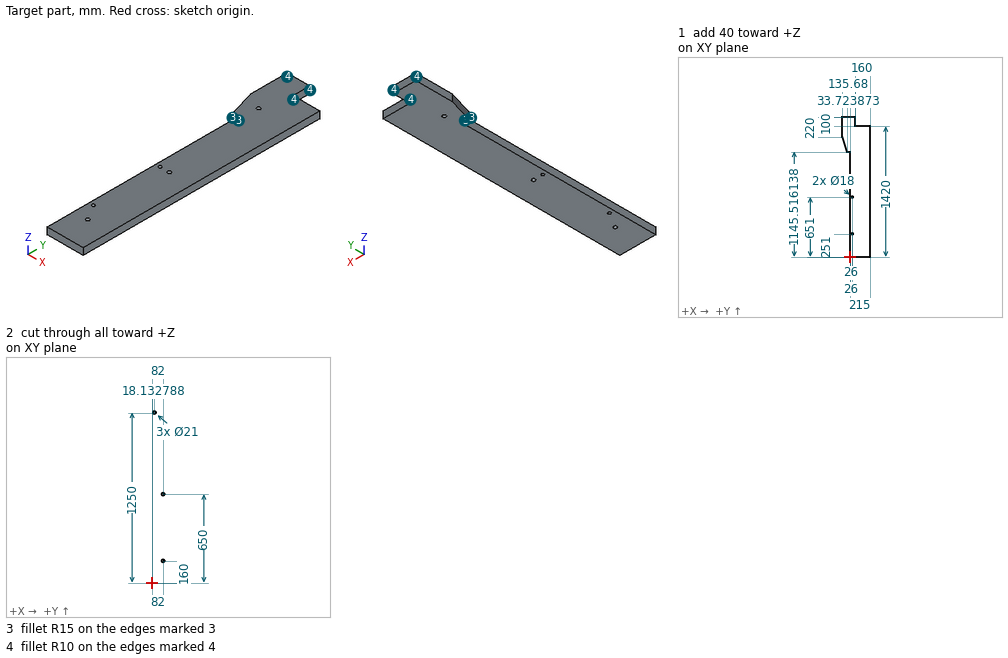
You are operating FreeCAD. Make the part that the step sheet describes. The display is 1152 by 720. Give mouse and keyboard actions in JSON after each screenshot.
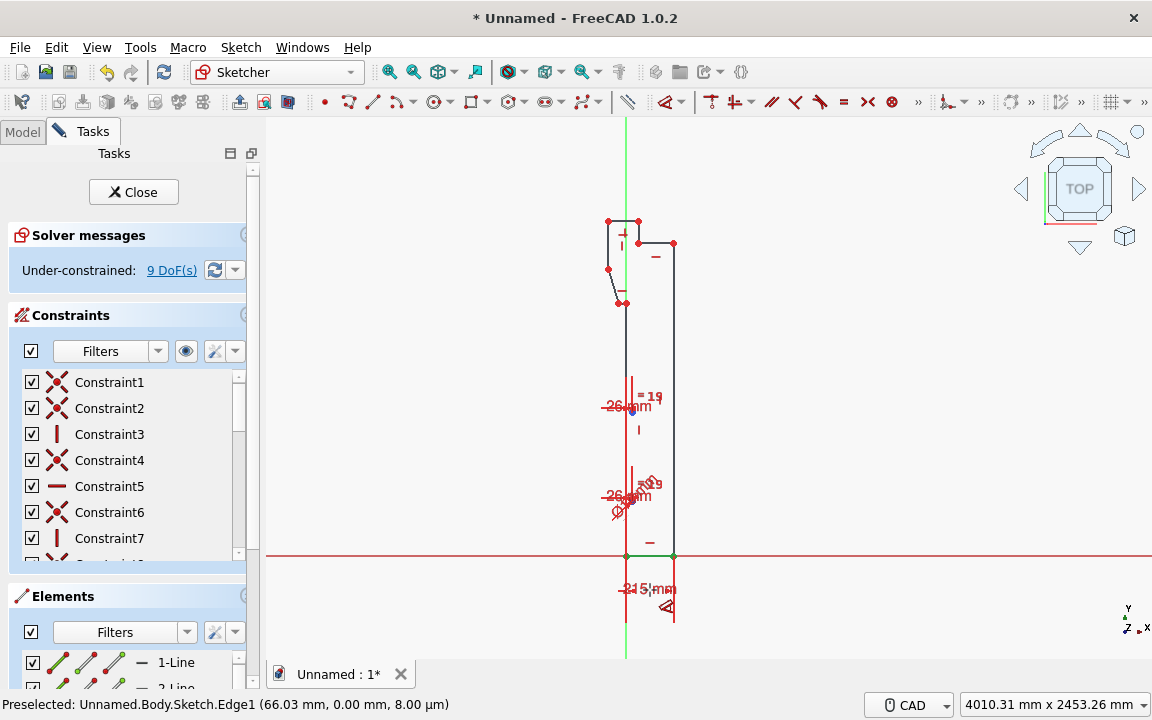
{"action": "scroll", "coordinate": [663, 243], "scroll_direction": "up", "scroll_amount": 2}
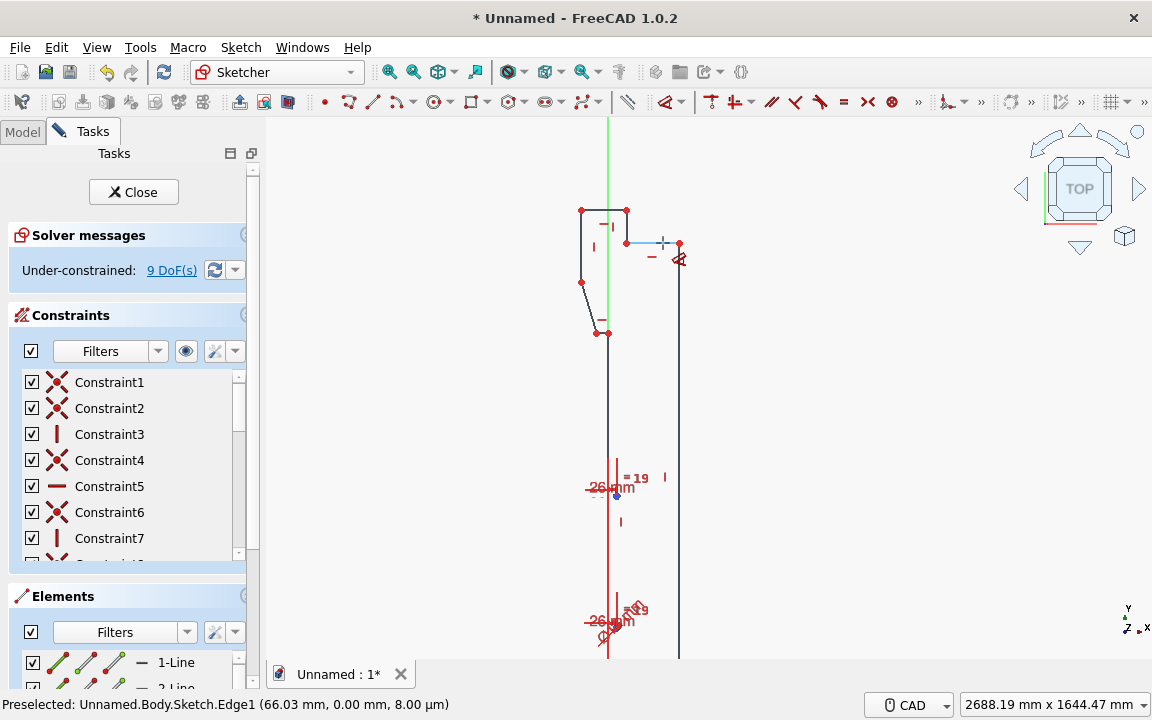
{"action": "left_click", "coordinate": [663, 243]}
{"action": "left_click", "coordinate": [653, 209]}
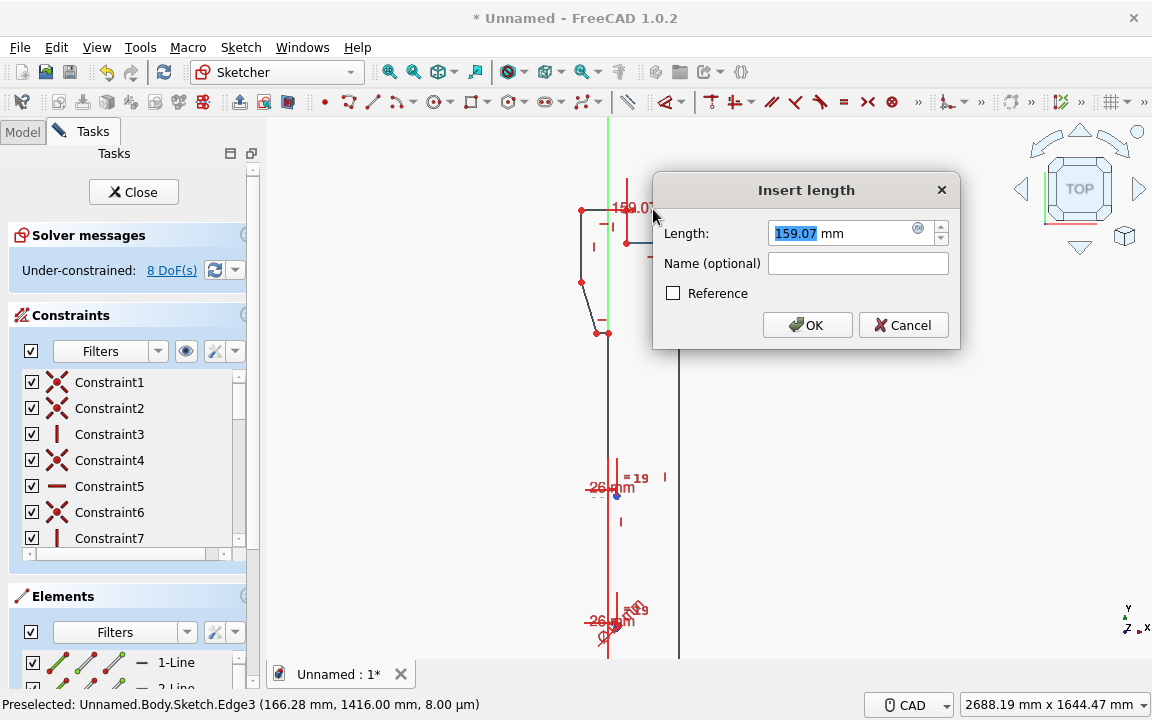
{"action": "type", "text": "160"}
{"action": "key", "text": "Return"}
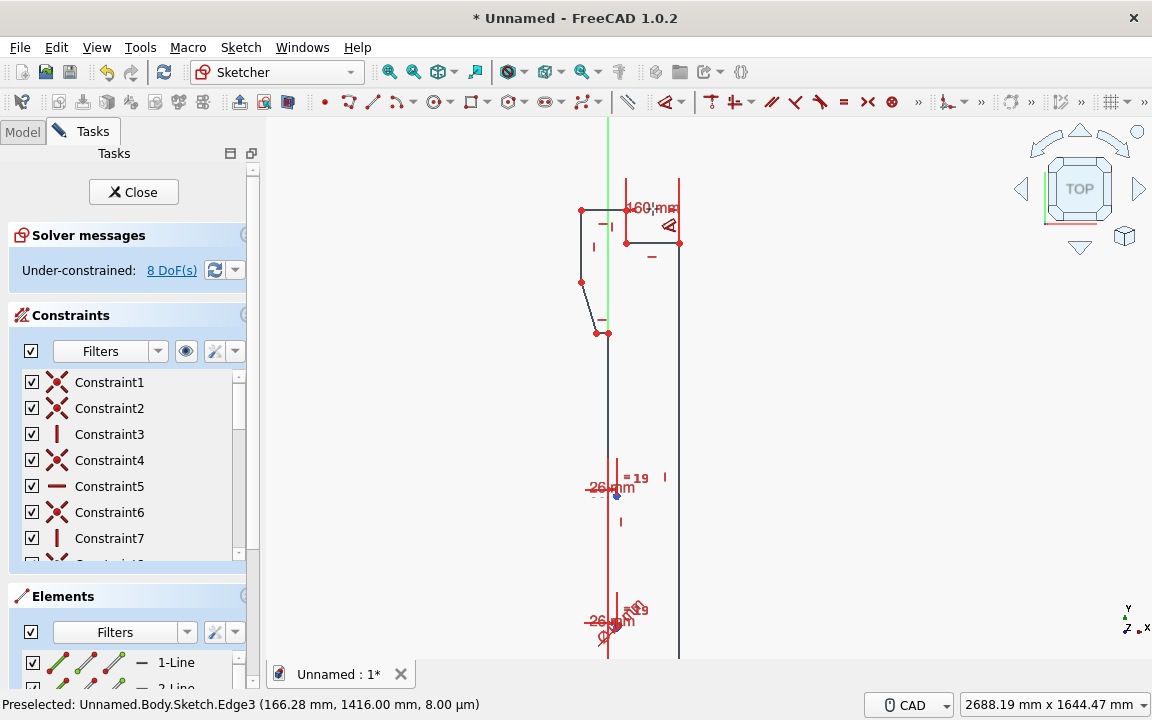
{"action": "scroll", "coordinate": [626, 233], "scroll_direction": "up", "scroll_amount": 2}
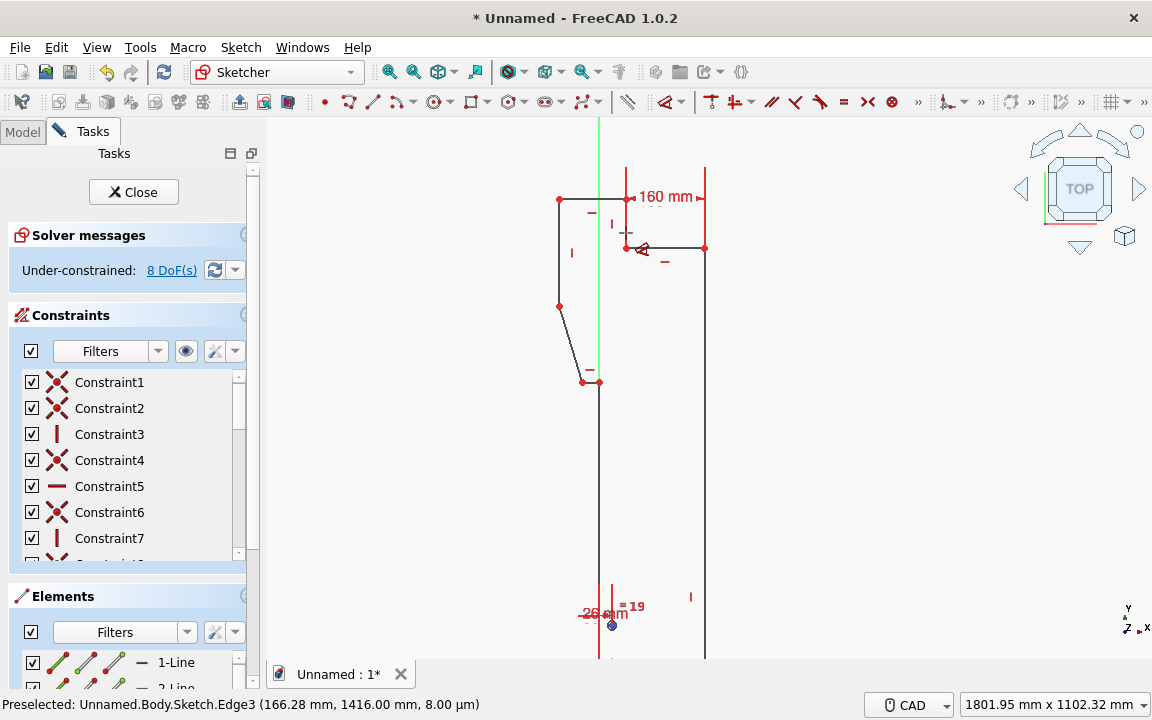
{"action": "left_click", "coordinate": [626, 234]}
{"action": "left_click", "coordinate": [660, 224]}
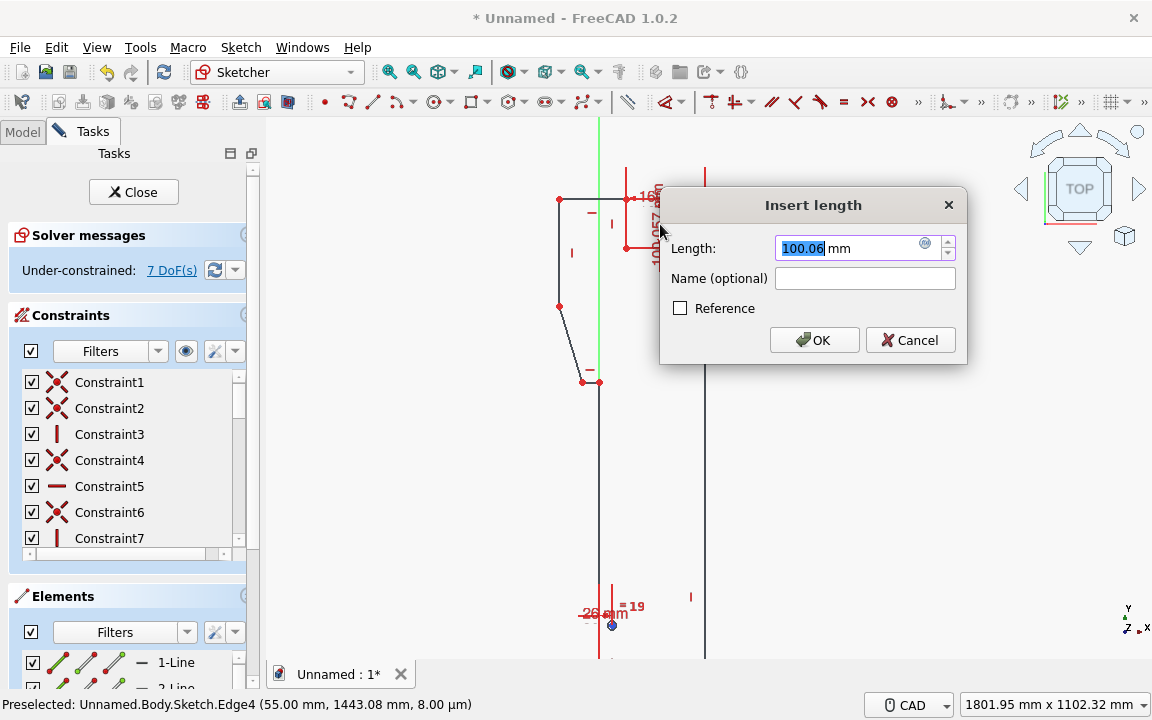
{"action": "type", "text": "100"}
{"action": "key", "text": "Return"}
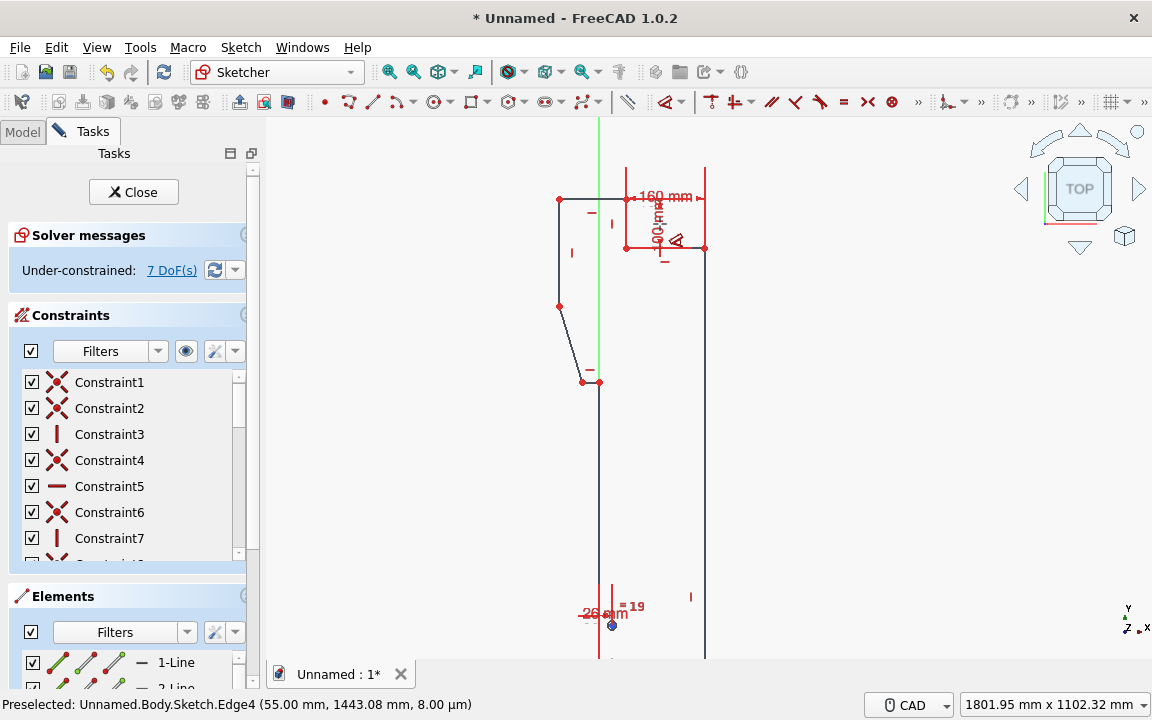
{"action": "left_click", "coordinate": [559, 231]}
{"action": "left_click", "coordinate": [525, 253]}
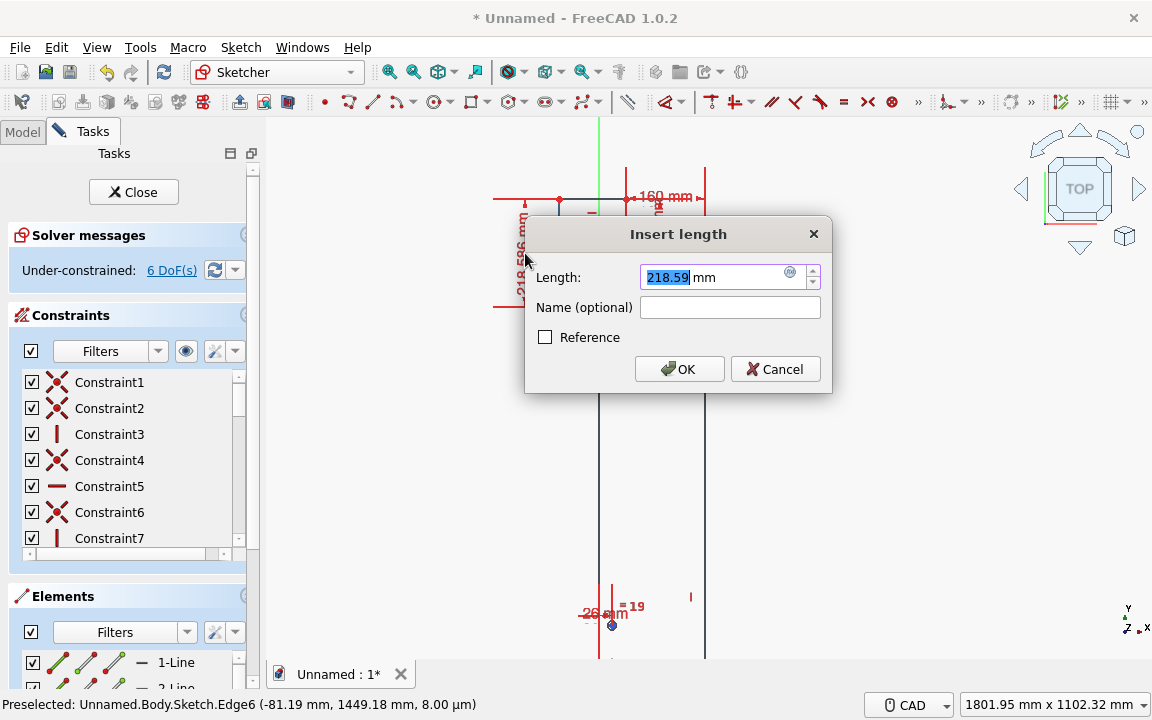
{"action": "type", "text": "220"}
{"action": "key", "text": "Return"}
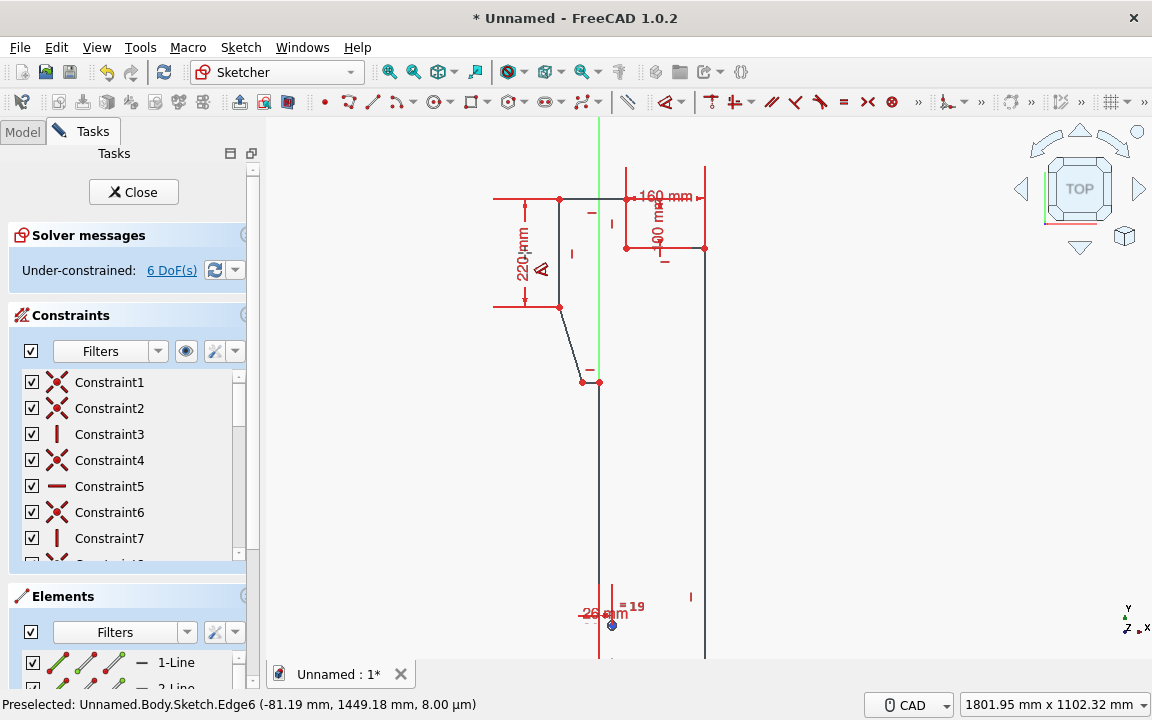
{"action": "scroll", "coordinate": [647, 239], "scroll_direction": "down", "scroll_amount": 4}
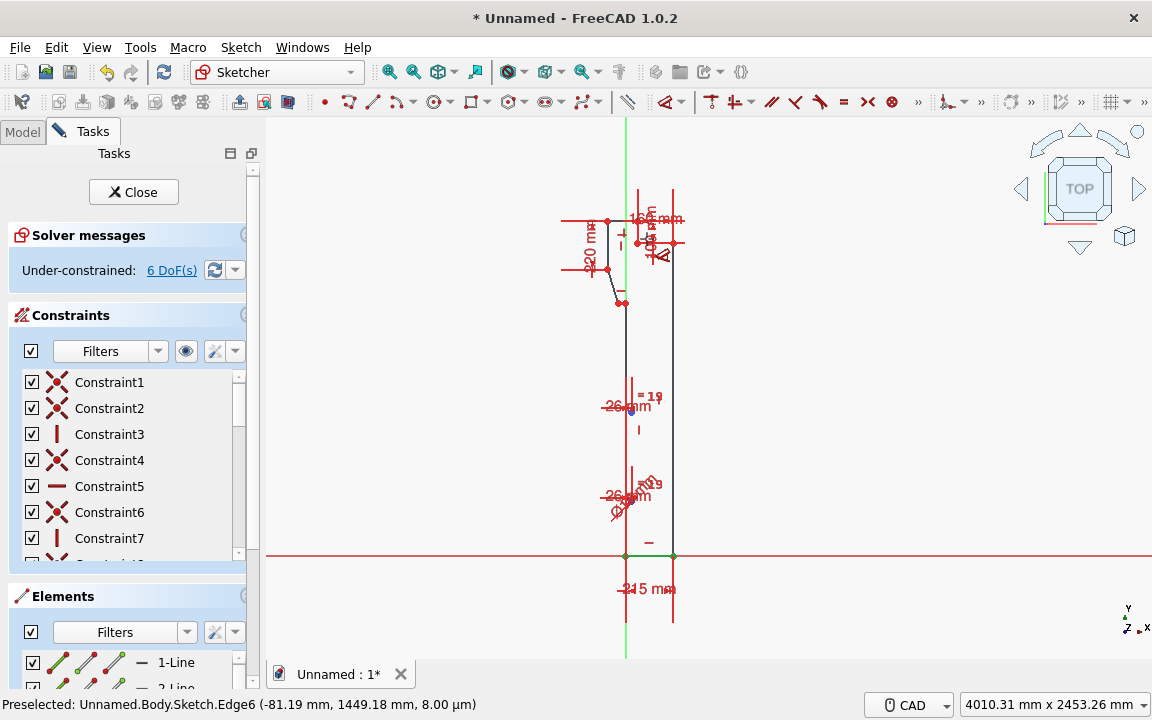
{"action": "left_click", "coordinate": [632, 501]}
{"action": "left_click", "coordinate": [592, 529]}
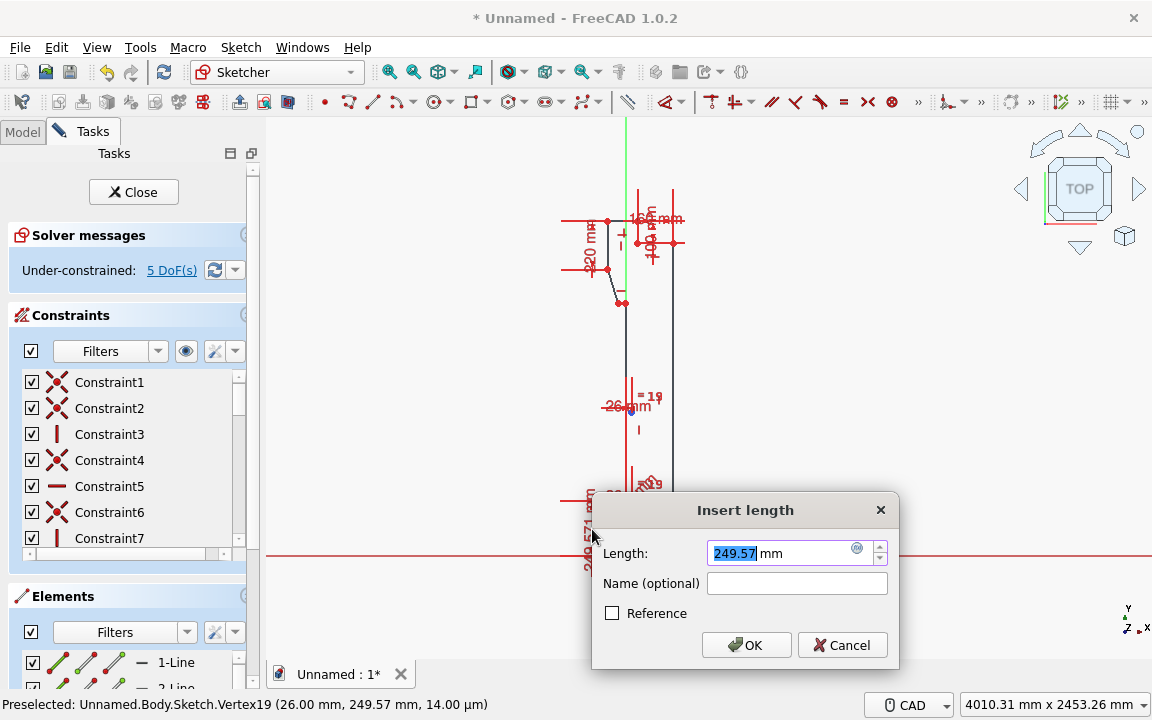
{"action": "type", "text": "251"}
{"action": "key", "text": "Return"}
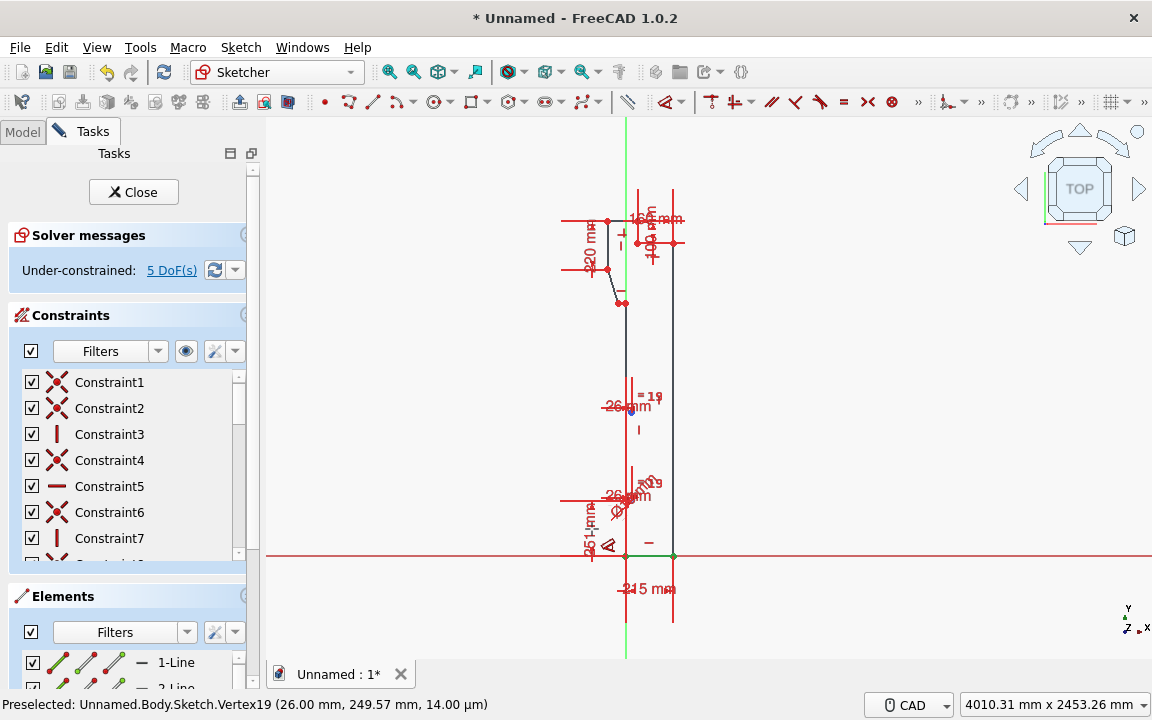
{"action": "left_click", "coordinate": [632, 413]}
{"action": "left_click", "coordinate": [592, 451]}